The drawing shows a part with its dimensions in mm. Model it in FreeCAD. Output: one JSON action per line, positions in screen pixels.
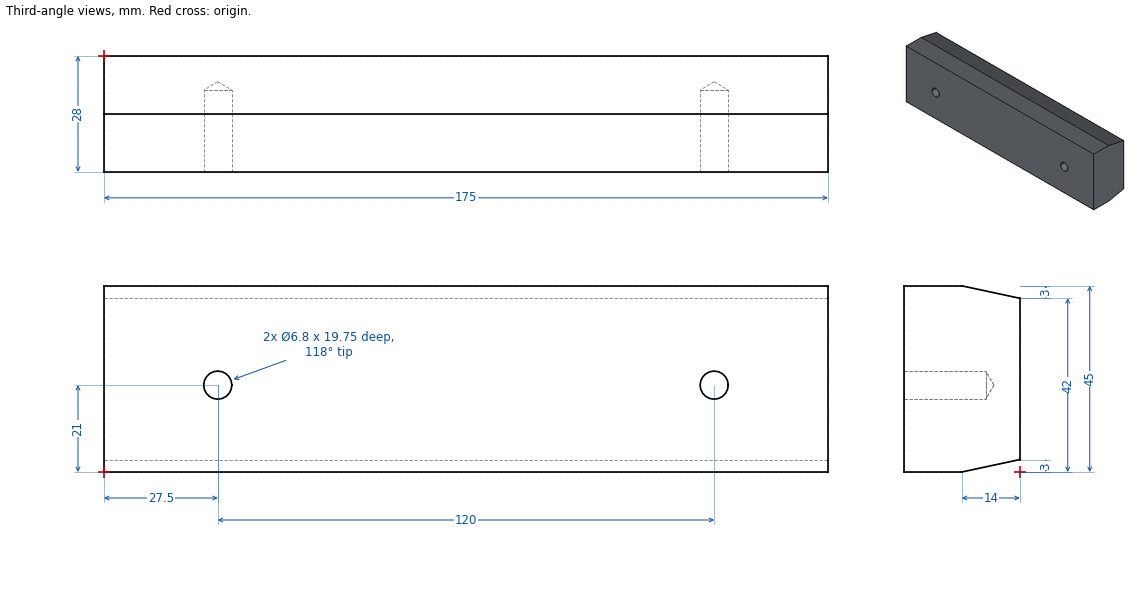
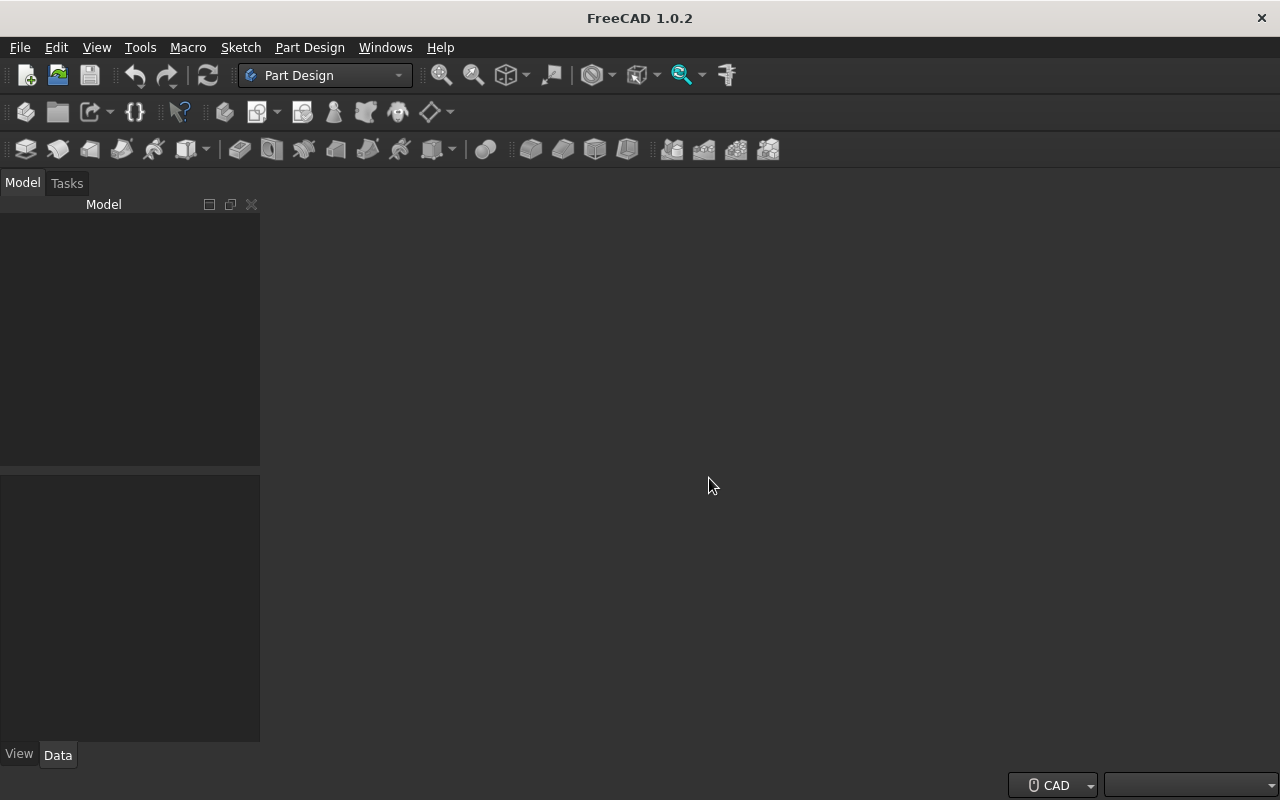
{"action": "left_click", "coordinate": [26, 76]}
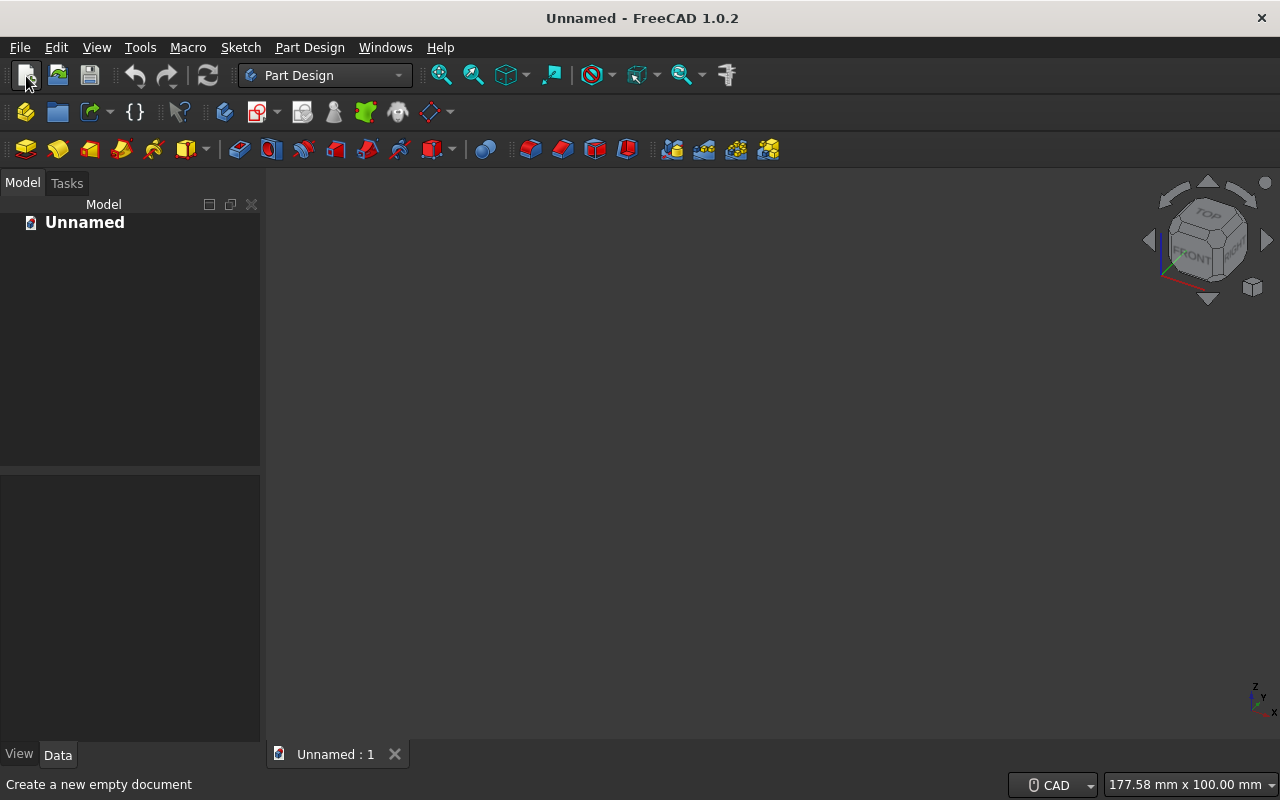
{"action": "left_click", "coordinate": [258, 112]}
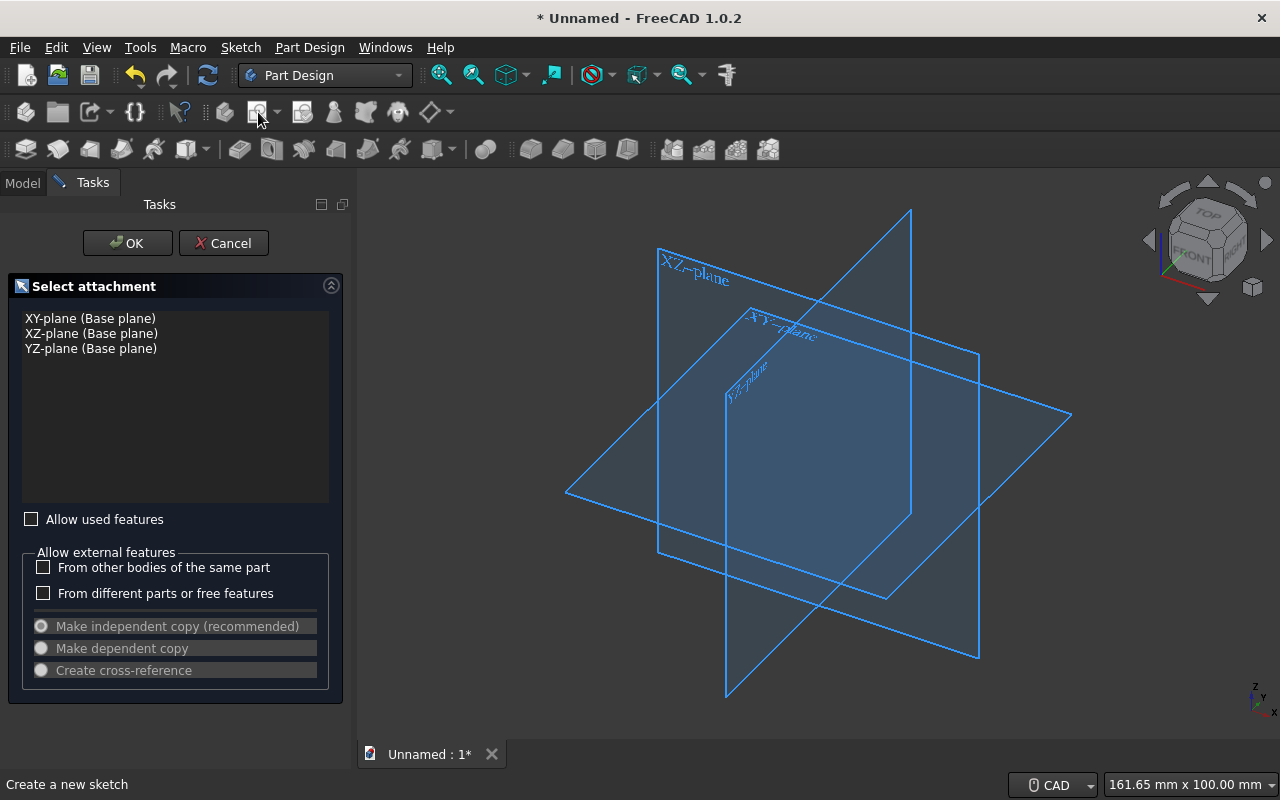
{"action": "left_click", "coordinate": [82, 318]}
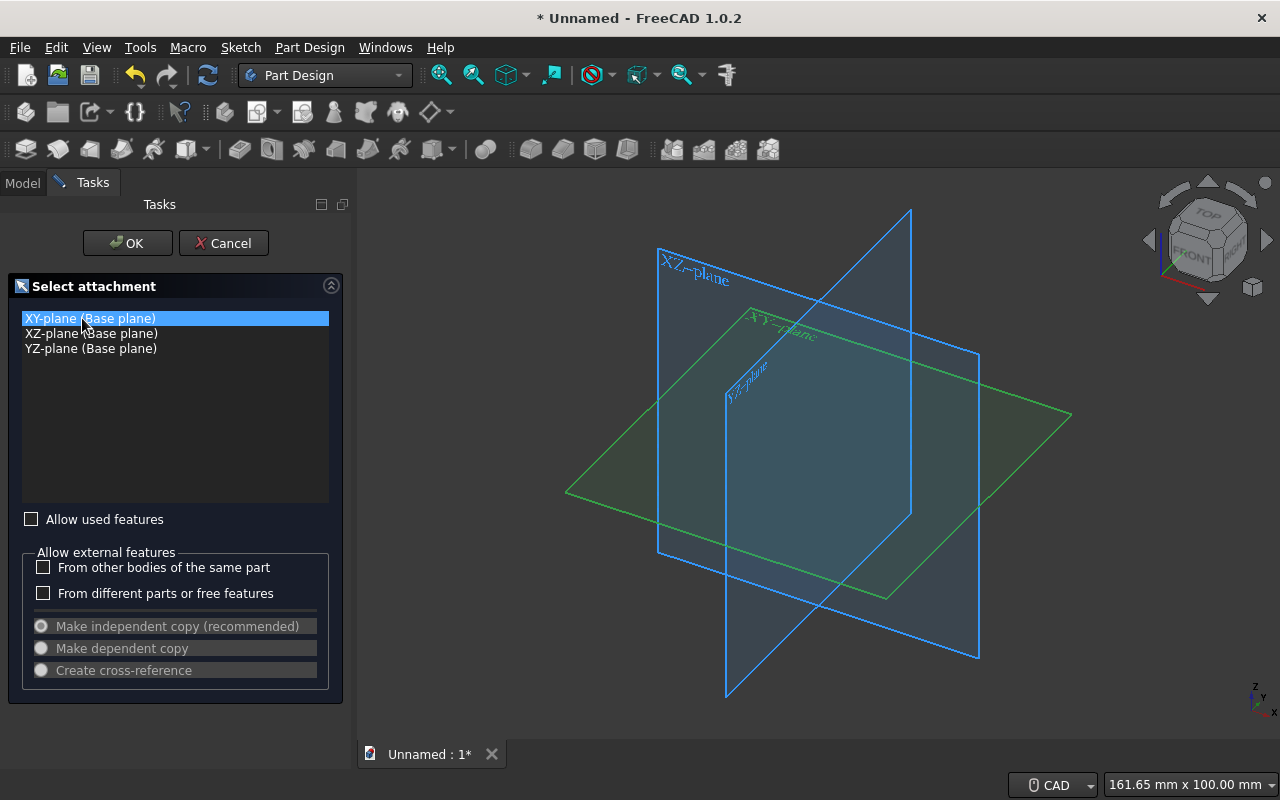
{"action": "left_click", "coordinate": [128, 243]}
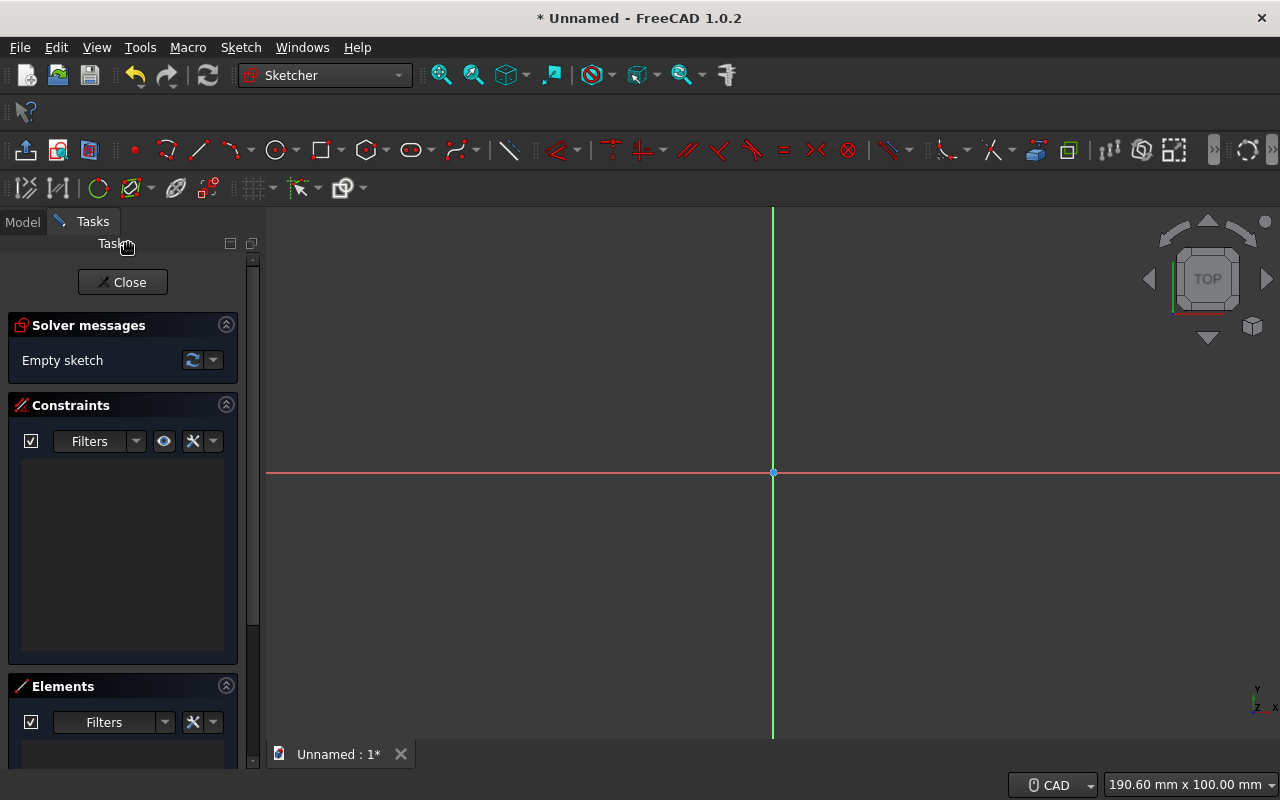
{"action": "scroll", "coordinate": [294, 382], "scroll_direction": "down", "scroll_amount": 3}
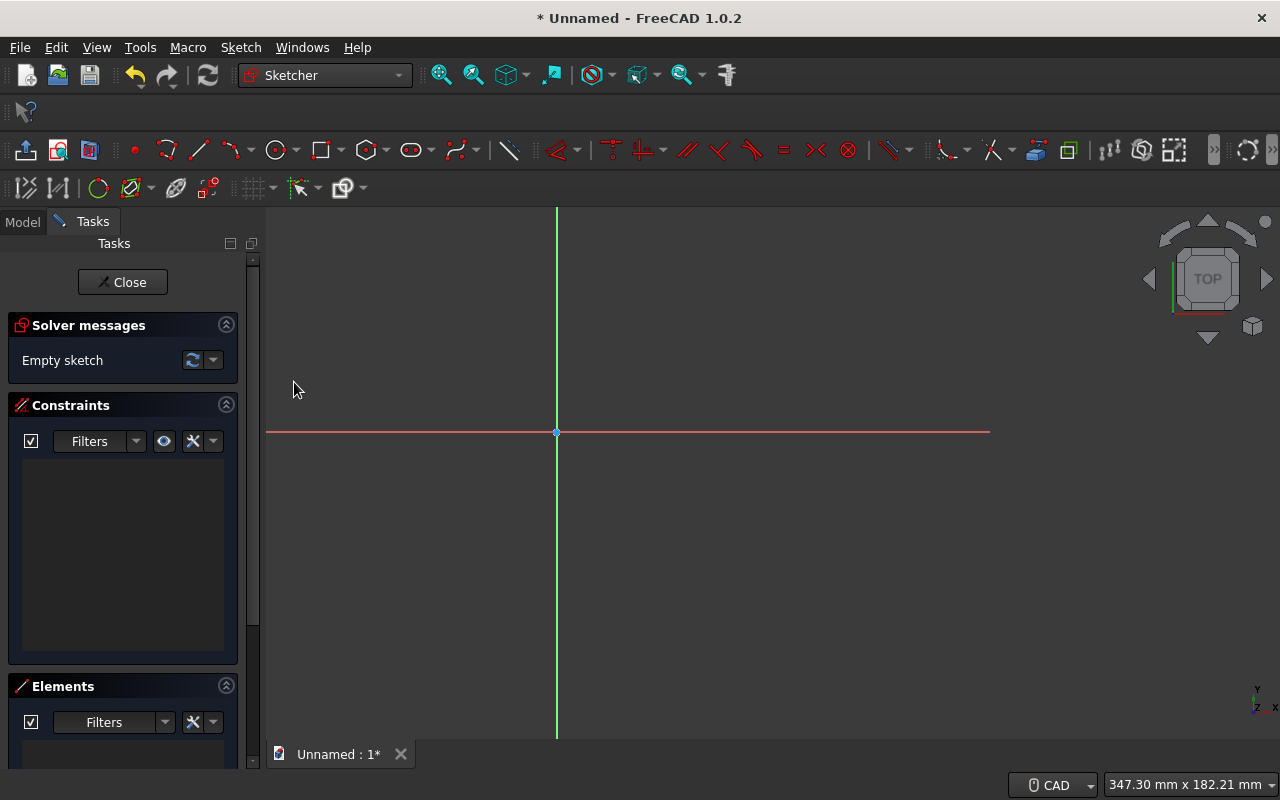
{"action": "key", "text": "g r"}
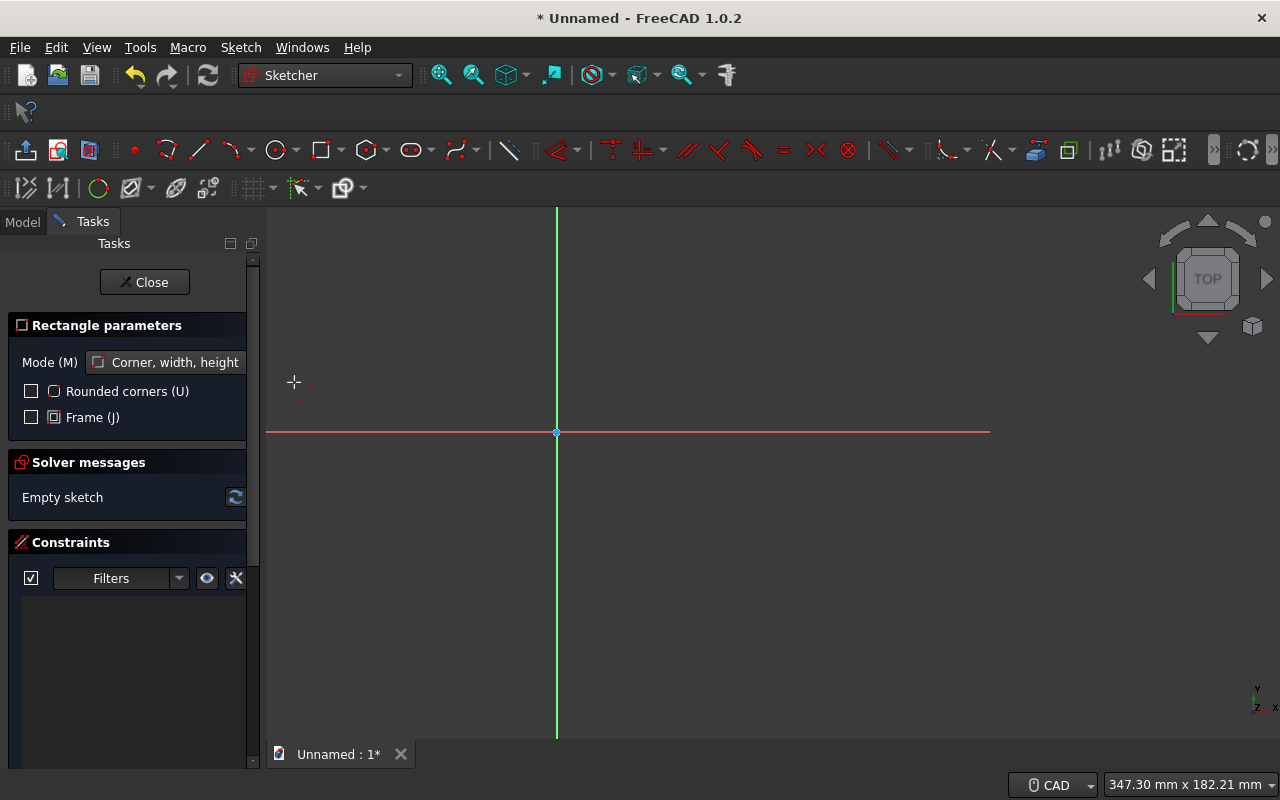
{"action": "left_click", "coordinate": [557, 432]}
{"action": "left_click", "coordinate": [1068, 514]}
{"action": "key", "text": "Escape"}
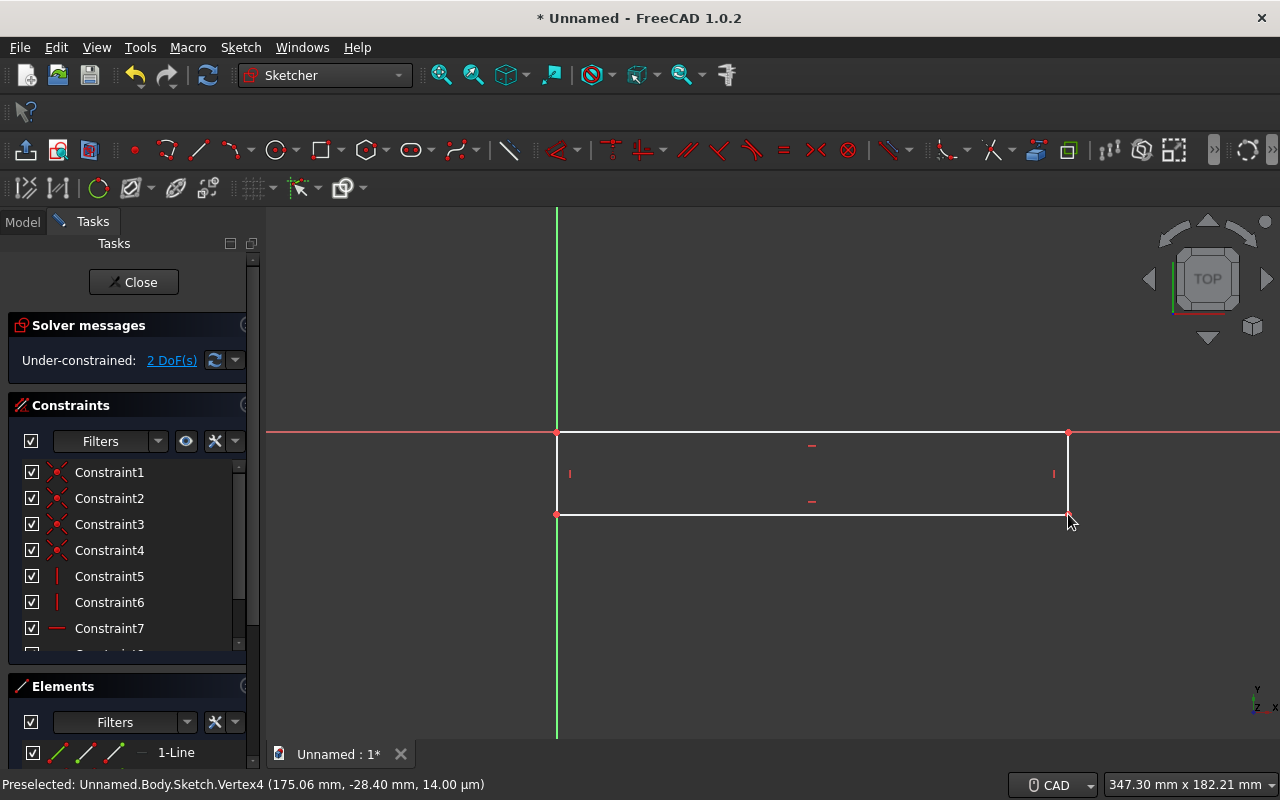
{"action": "left_click", "coordinate": [556, 150]}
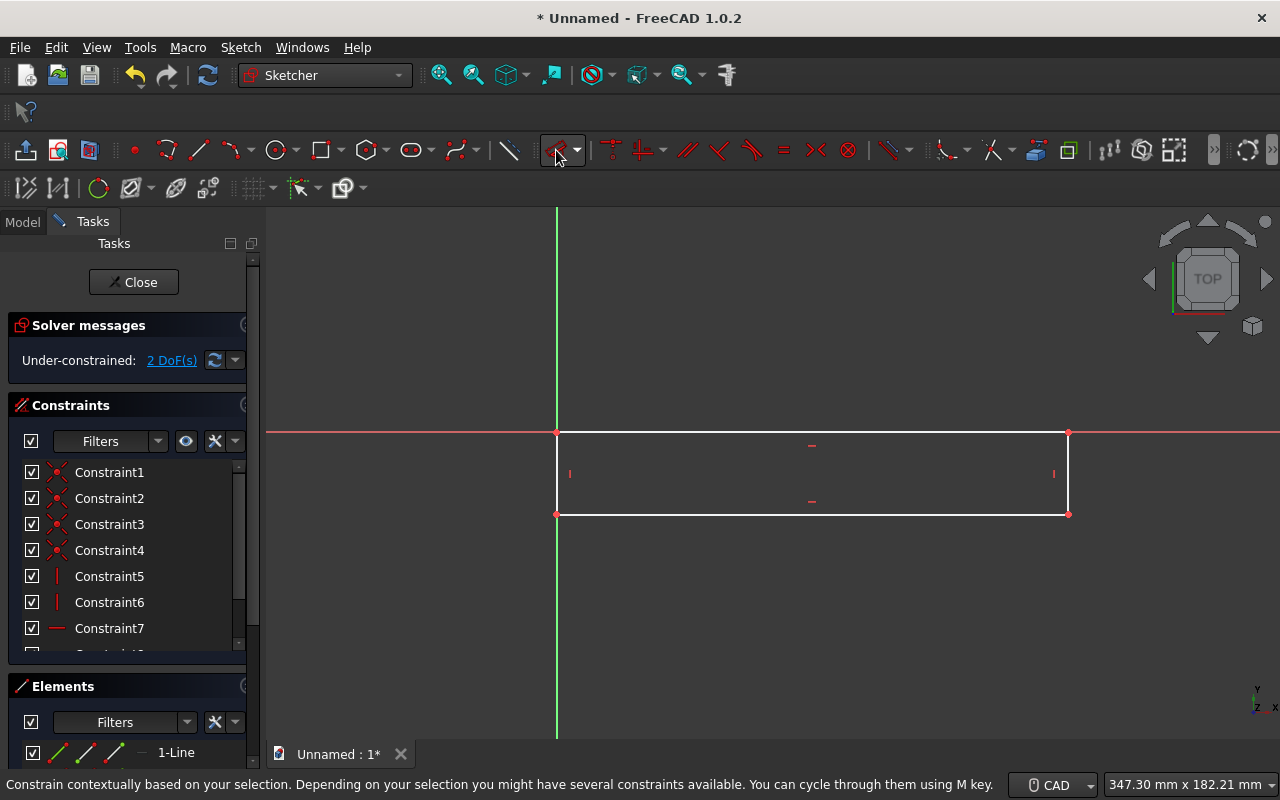
{"action": "left_click", "coordinate": [557, 457]}
{"action": "left_click", "coordinate": [523, 474]}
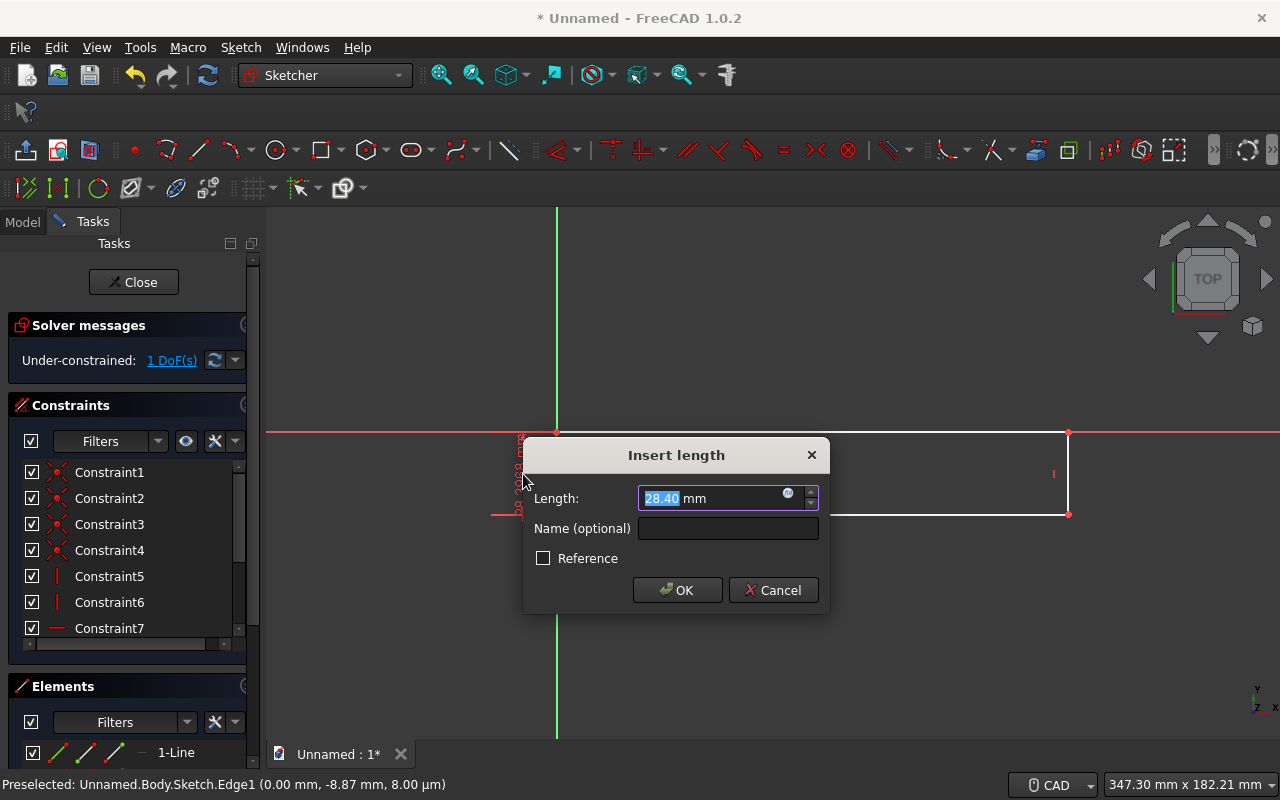
{"action": "type", "text": "28"}
{"action": "key", "text": "Return"}